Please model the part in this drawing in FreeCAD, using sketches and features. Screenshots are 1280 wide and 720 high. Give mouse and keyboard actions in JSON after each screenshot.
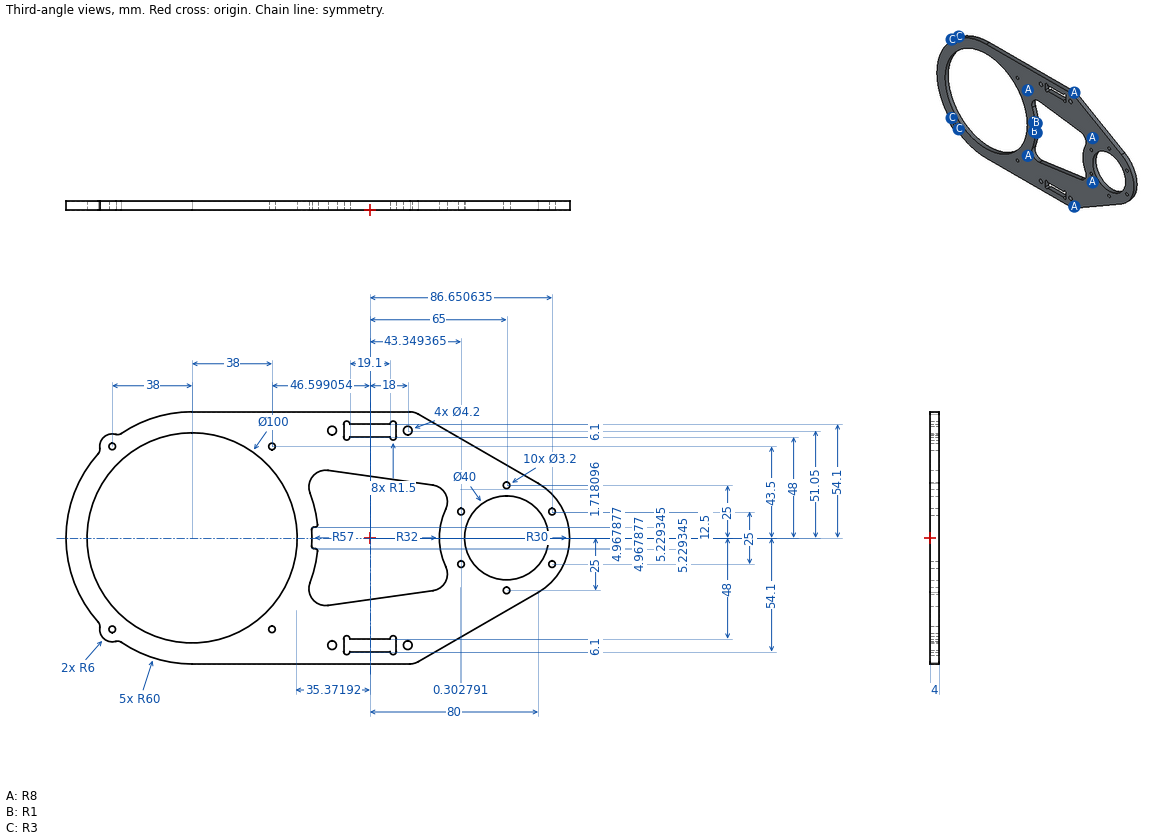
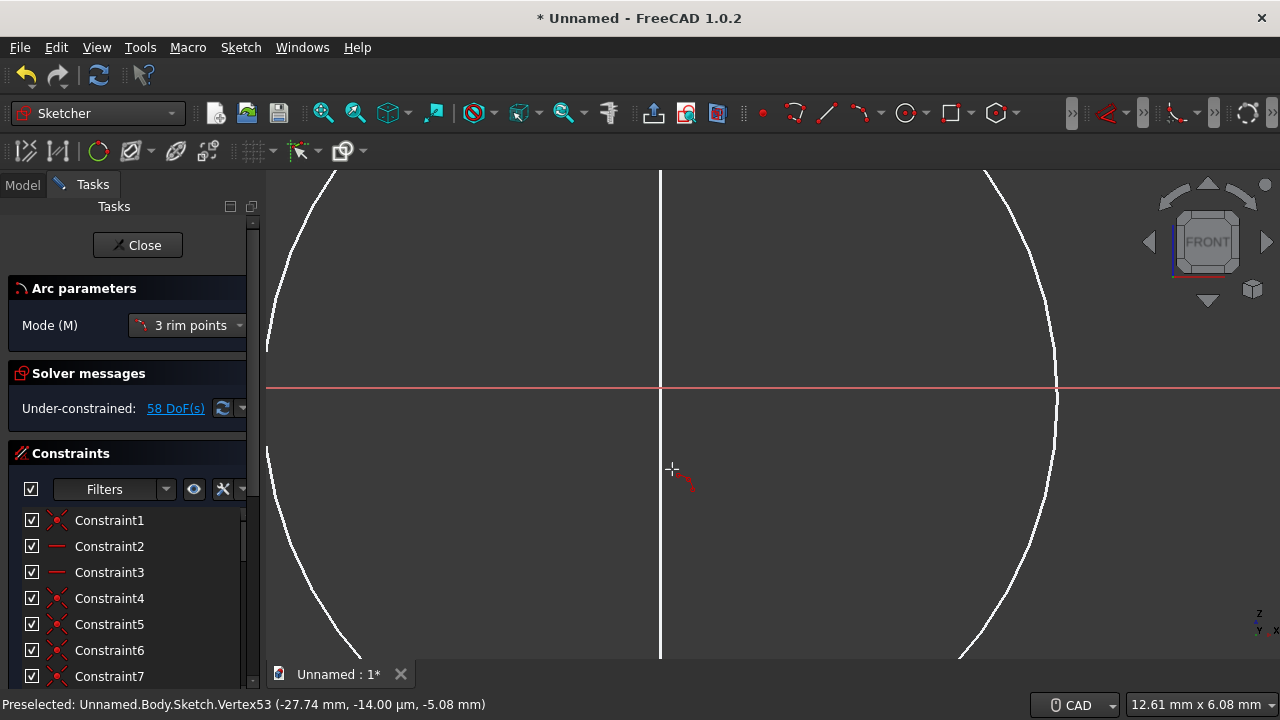
{"action": "left_click", "coordinate": [671, 468]}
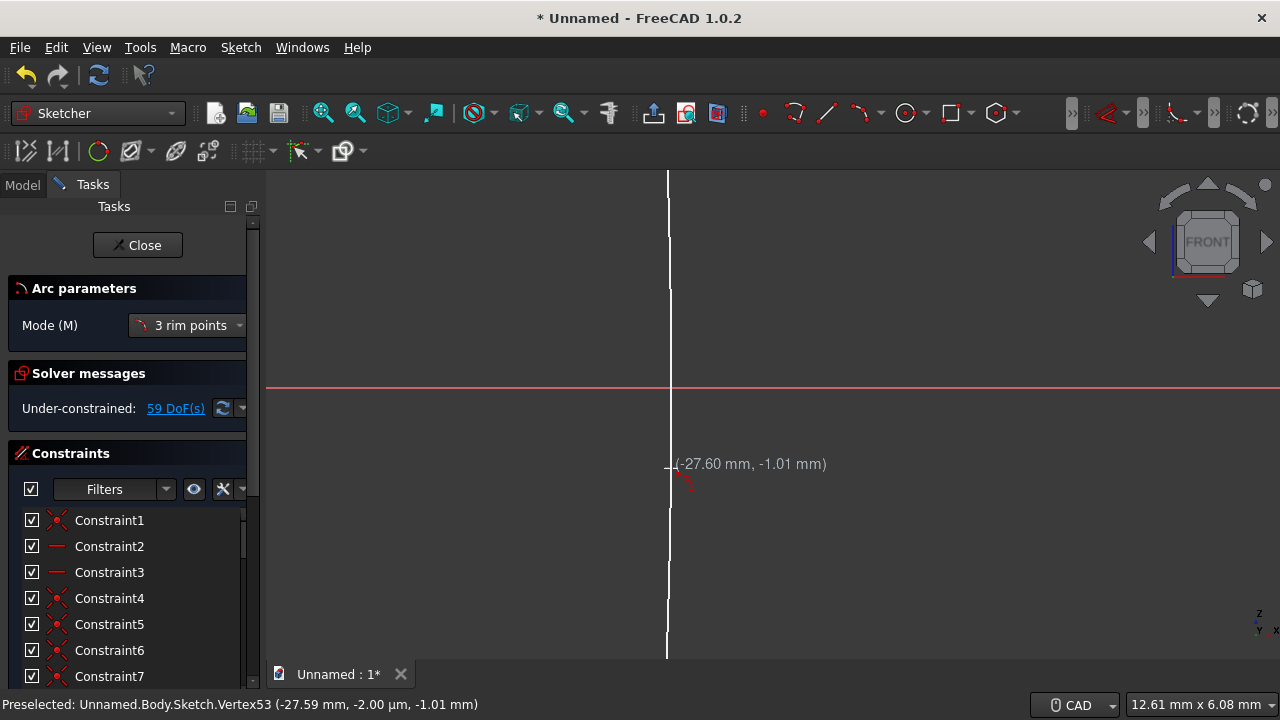
{"action": "scroll", "coordinate": [698, 415], "scroll_direction": "down", "scroll_amount": 17}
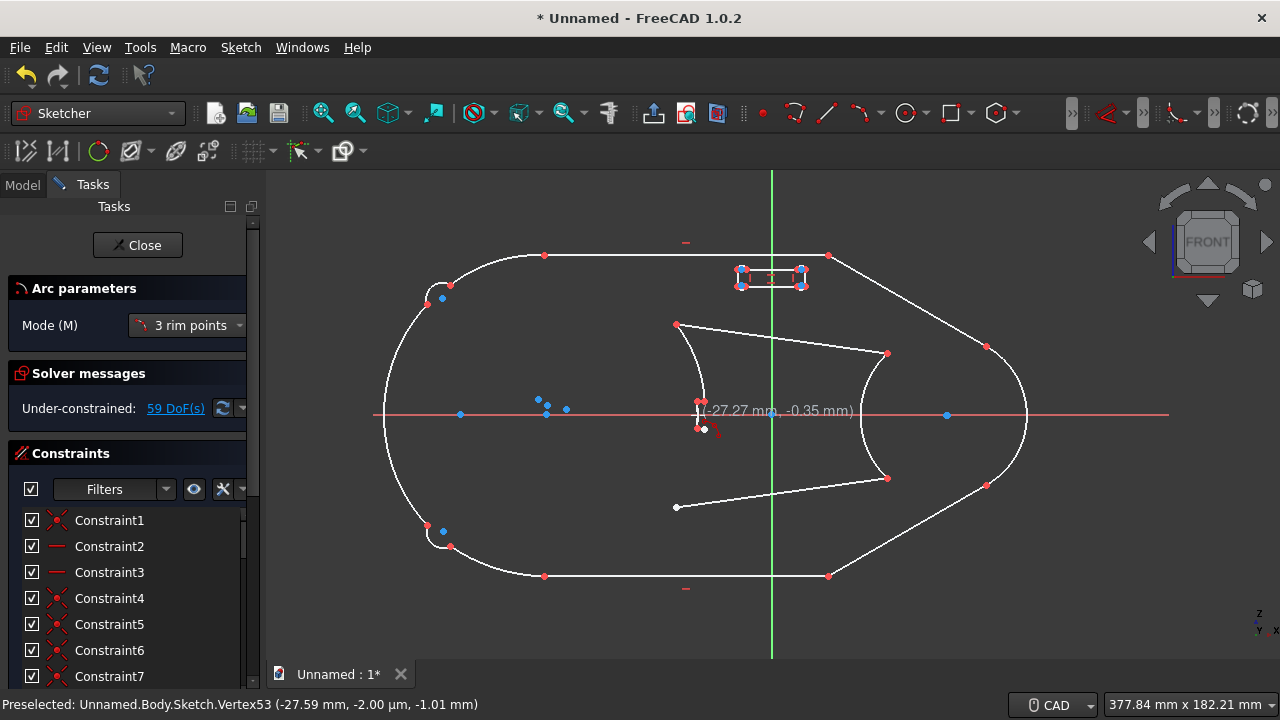
{"action": "scroll", "coordinate": [705, 429], "scroll_direction": "up", "scroll_amount": 7}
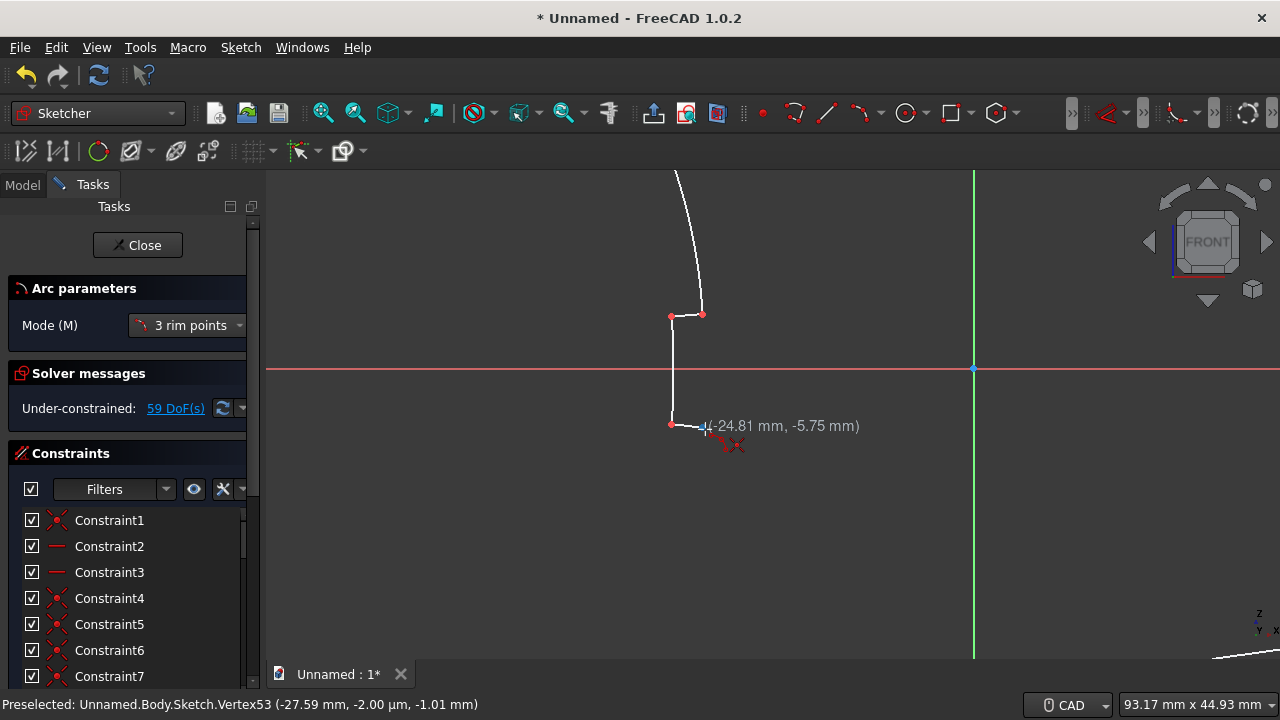
{"action": "left_click", "coordinate": [703, 428]}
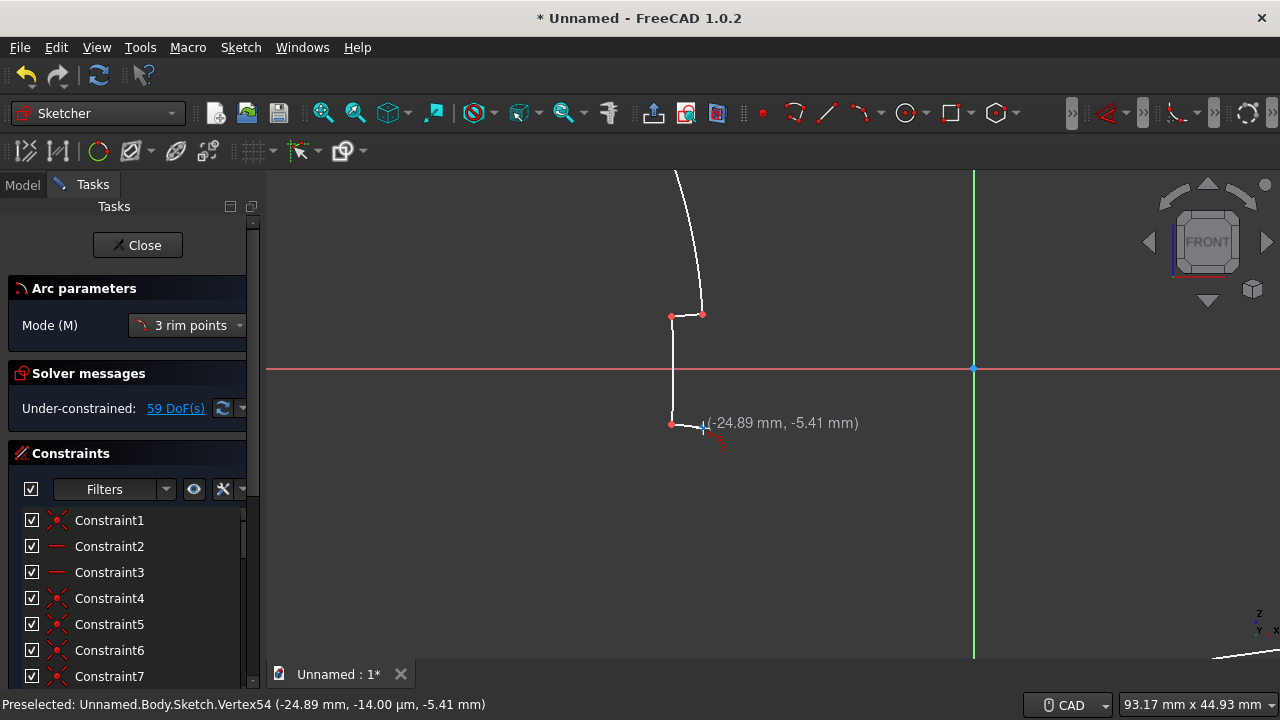
{"action": "scroll", "coordinate": [705, 426], "scroll_direction": "down", "scroll_amount": 8}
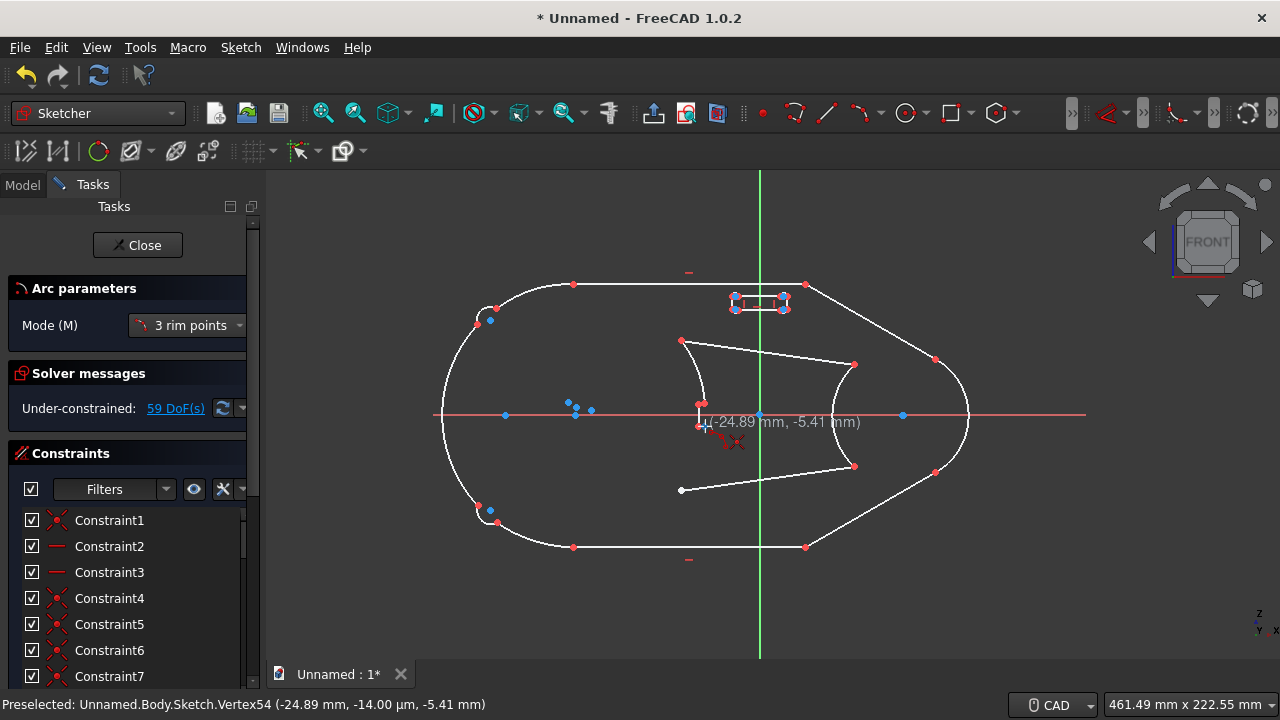
{"action": "left_click", "coordinate": [681, 491]}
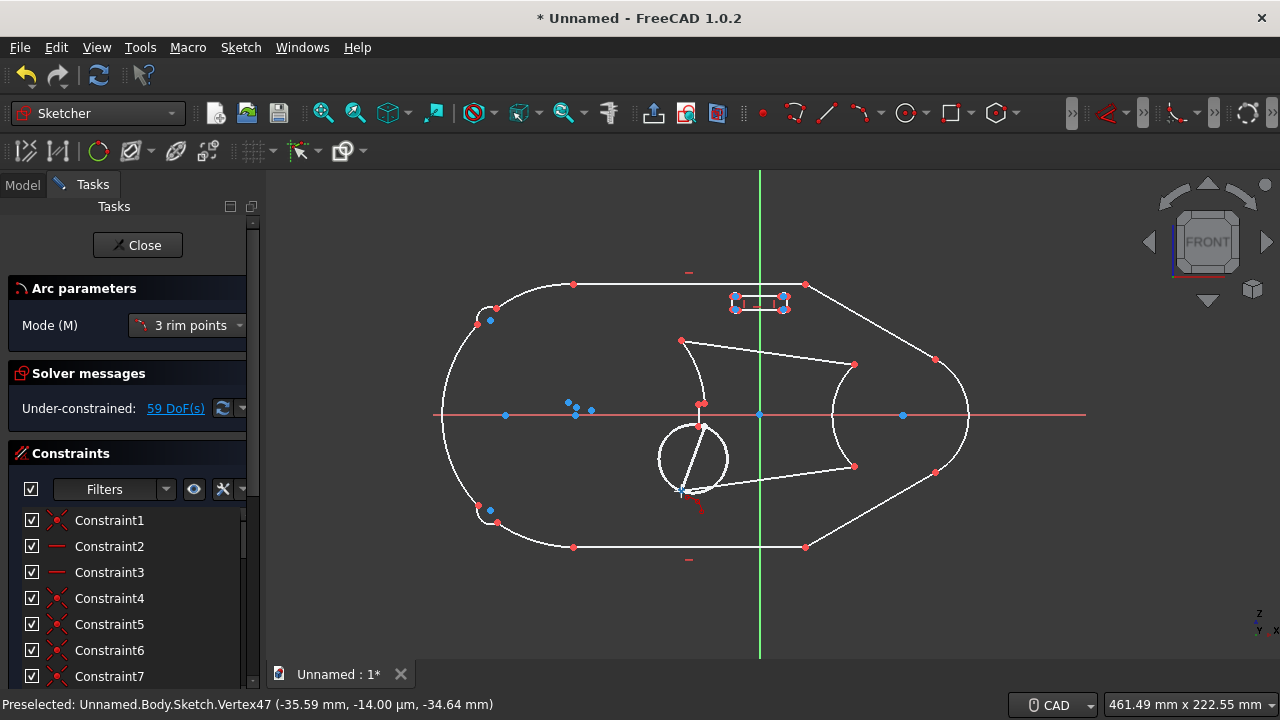
{"action": "scroll", "coordinate": [698, 460], "scroll_direction": "up", "scroll_amount": 7}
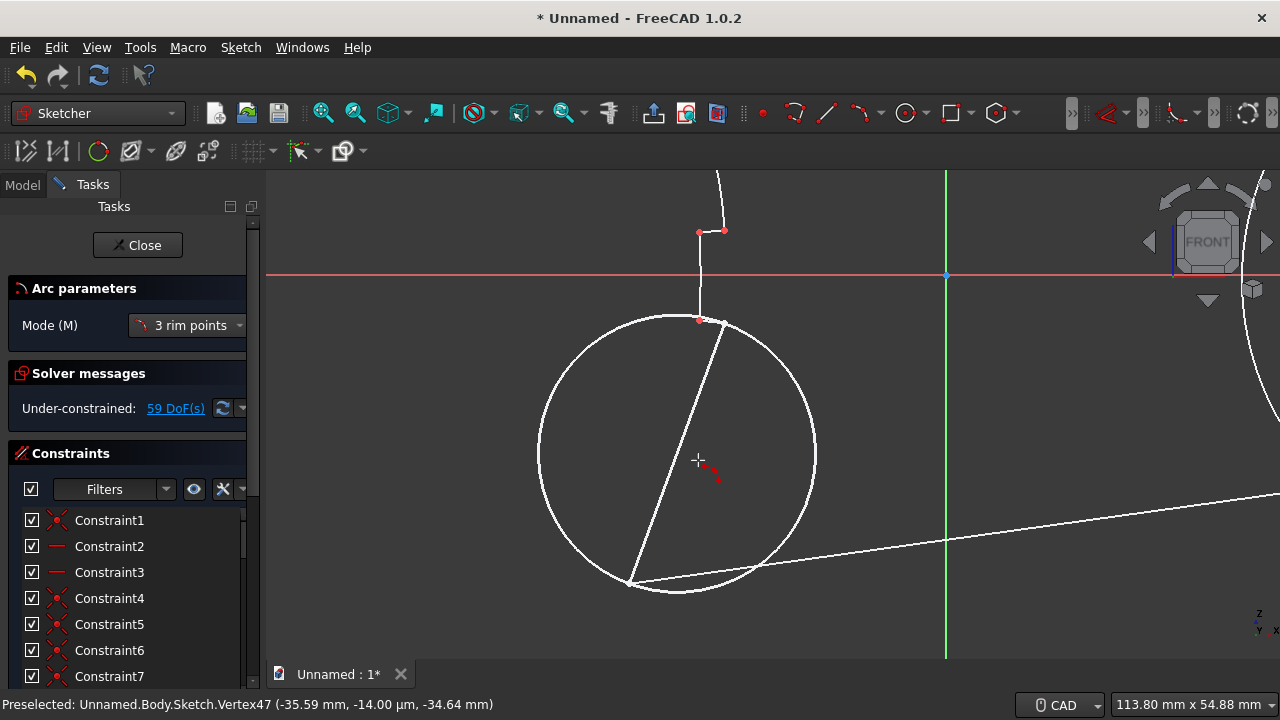
{"action": "left_click", "coordinate": [695, 458]}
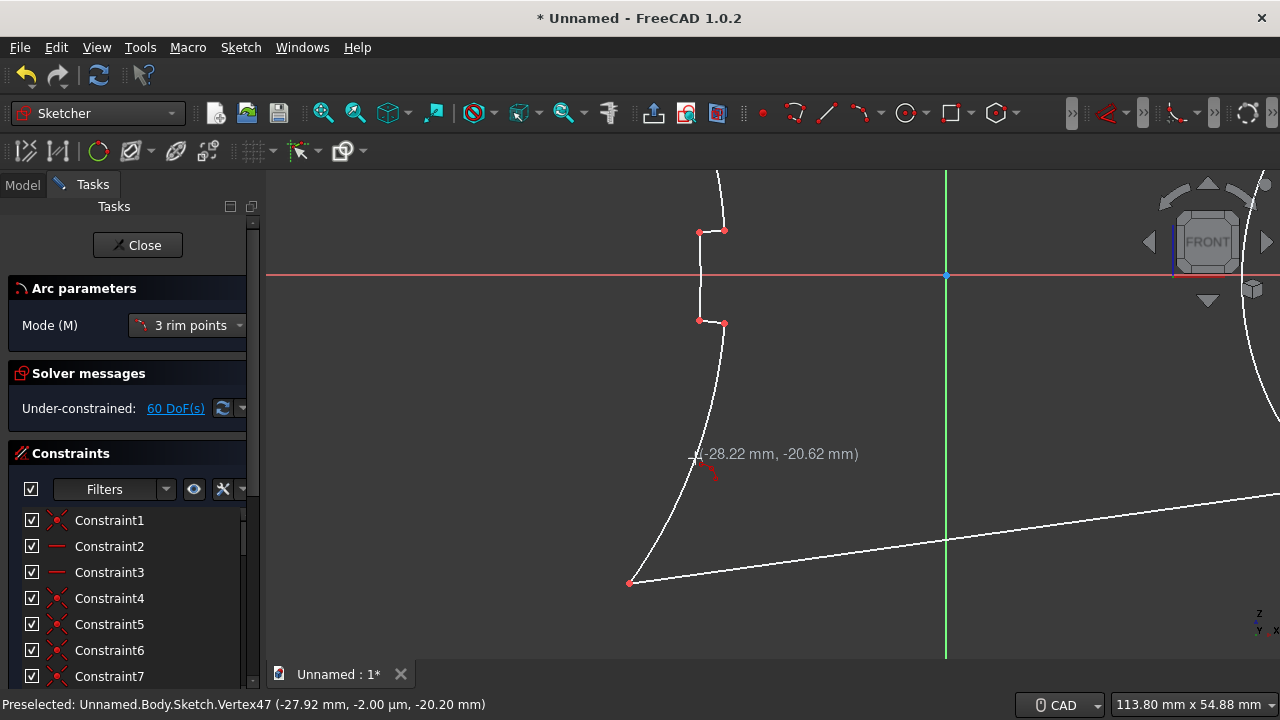
{"action": "left_click", "coordinate": [828, 114]}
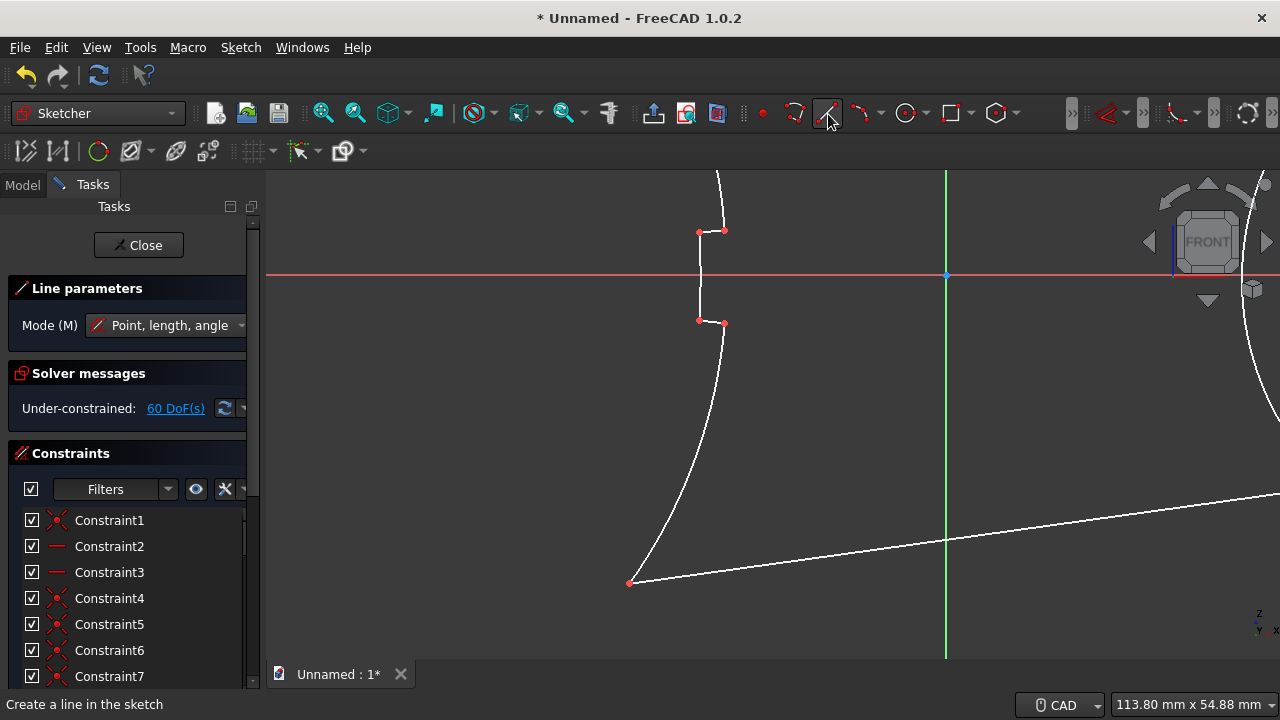
{"action": "scroll", "coordinate": [698, 460], "scroll_direction": "down", "scroll_amount": 7}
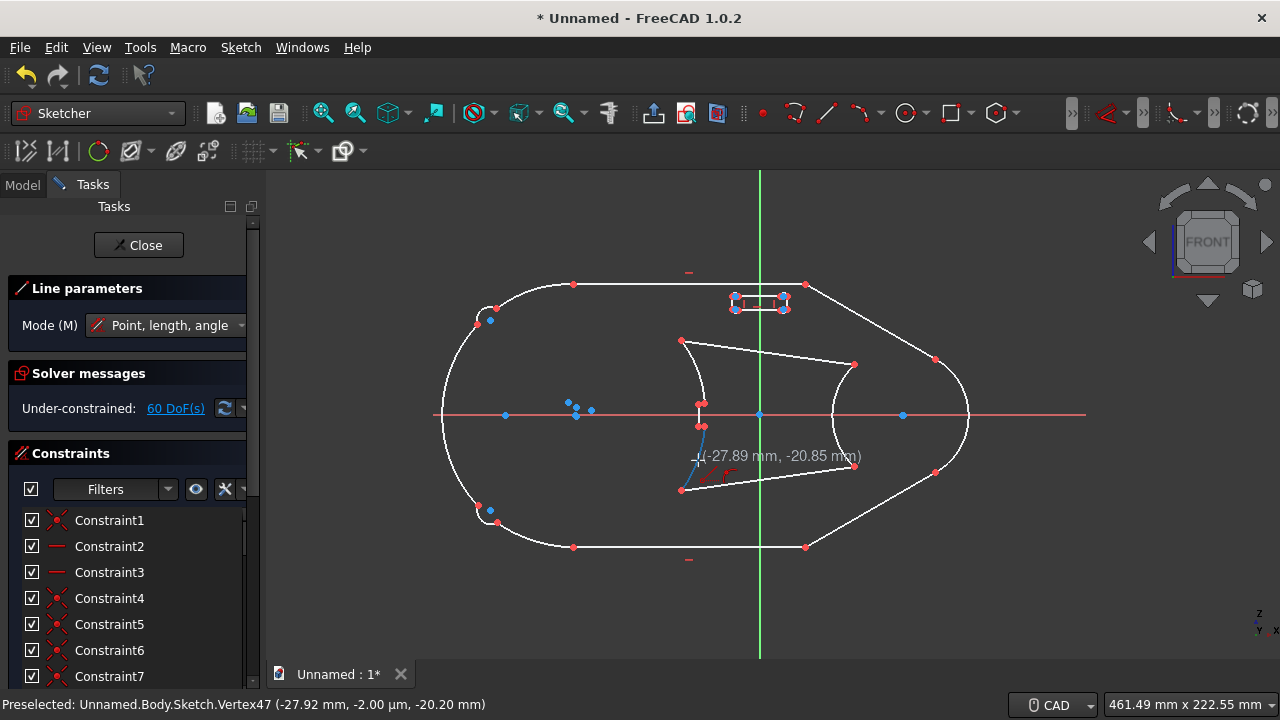
{"action": "scroll", "coordinate": [739, 534], "scroll_direction": "up", "scroll_amount": 2}